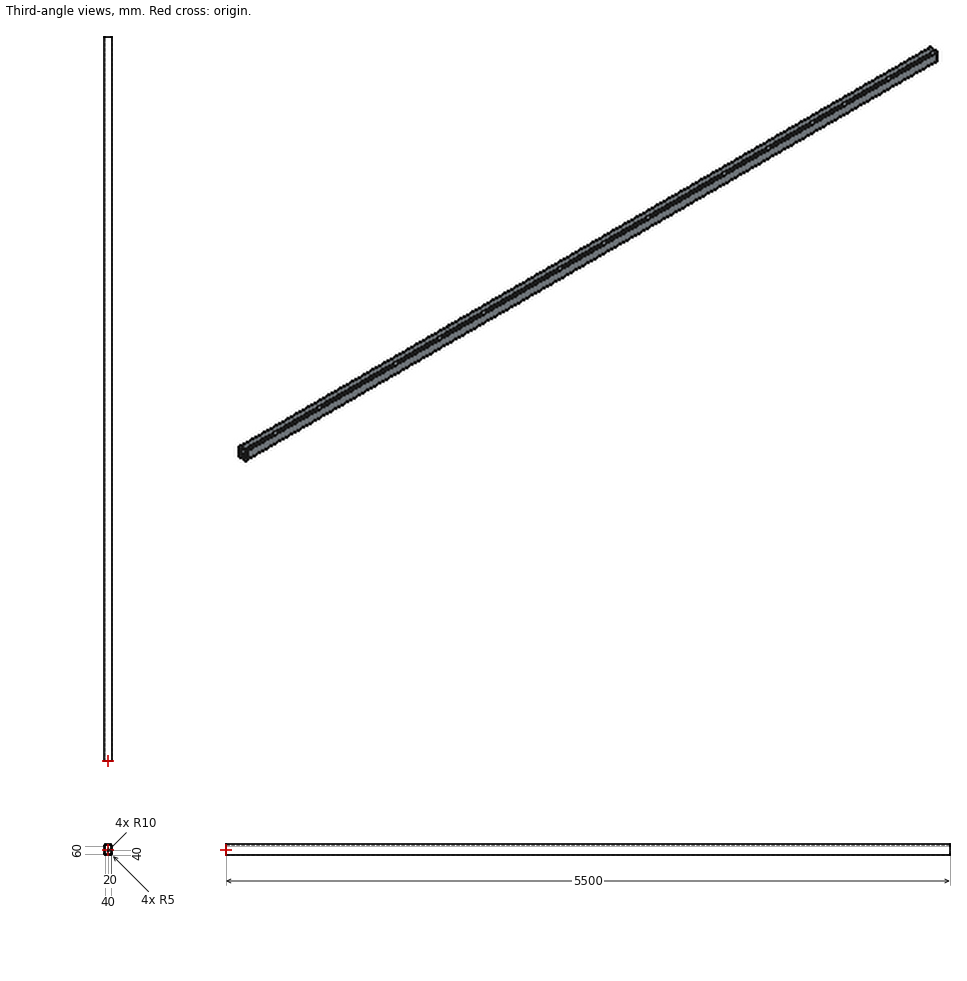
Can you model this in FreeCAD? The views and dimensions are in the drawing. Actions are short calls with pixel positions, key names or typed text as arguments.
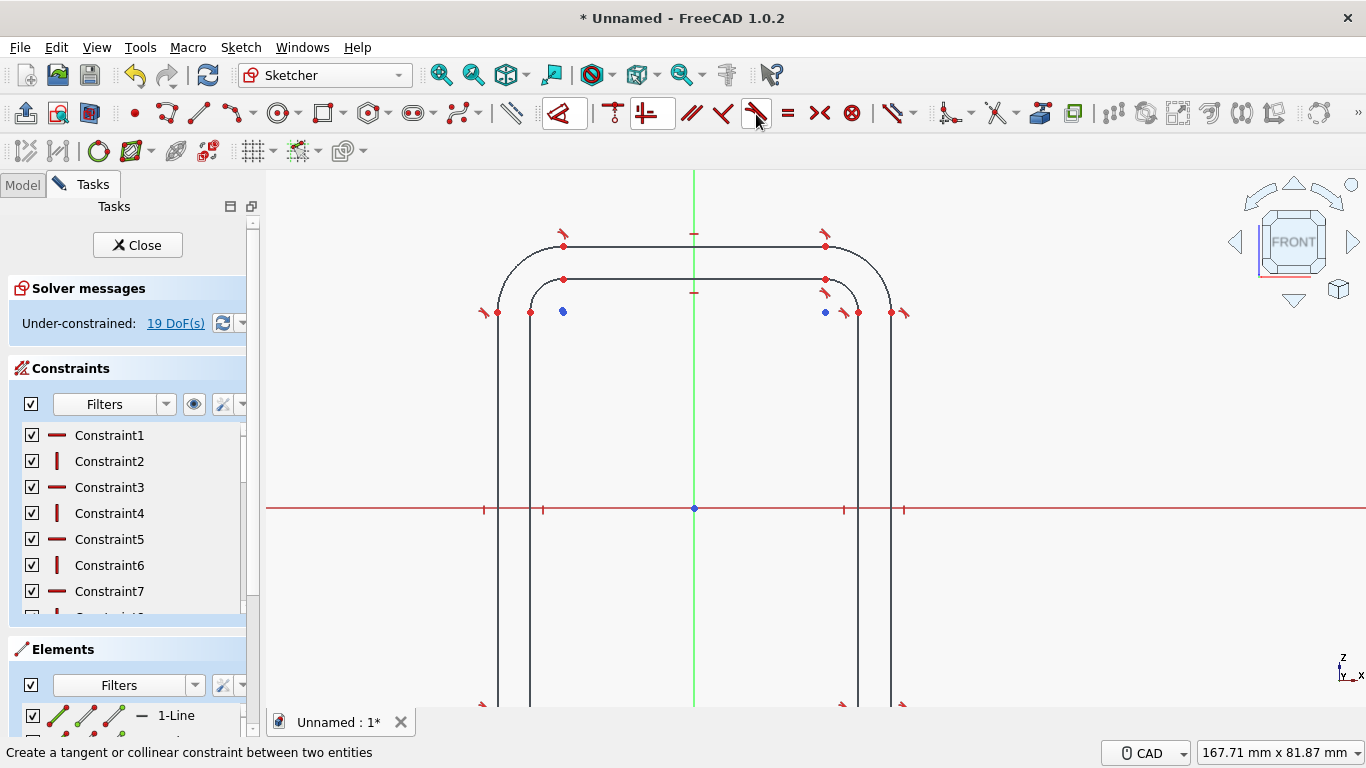
click(747, 279)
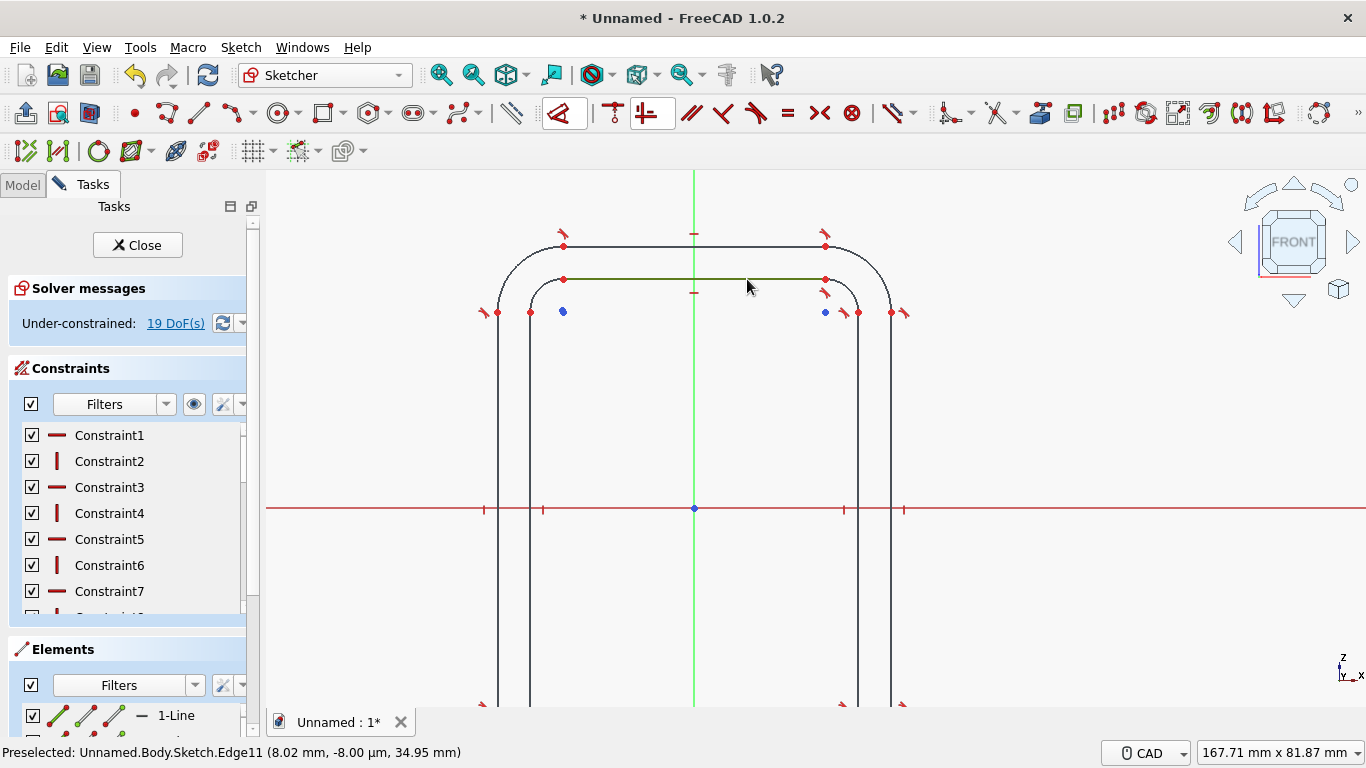
click(548, 282)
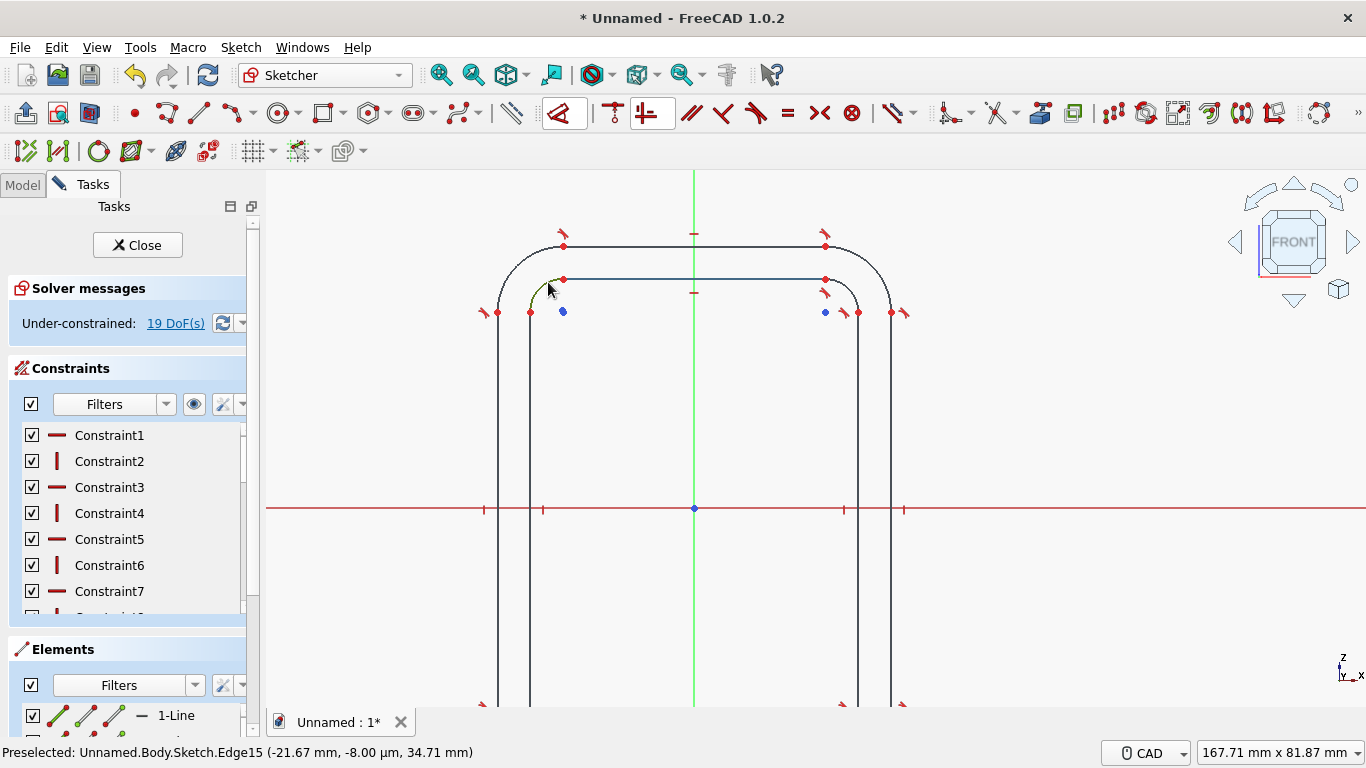
click(756, 114)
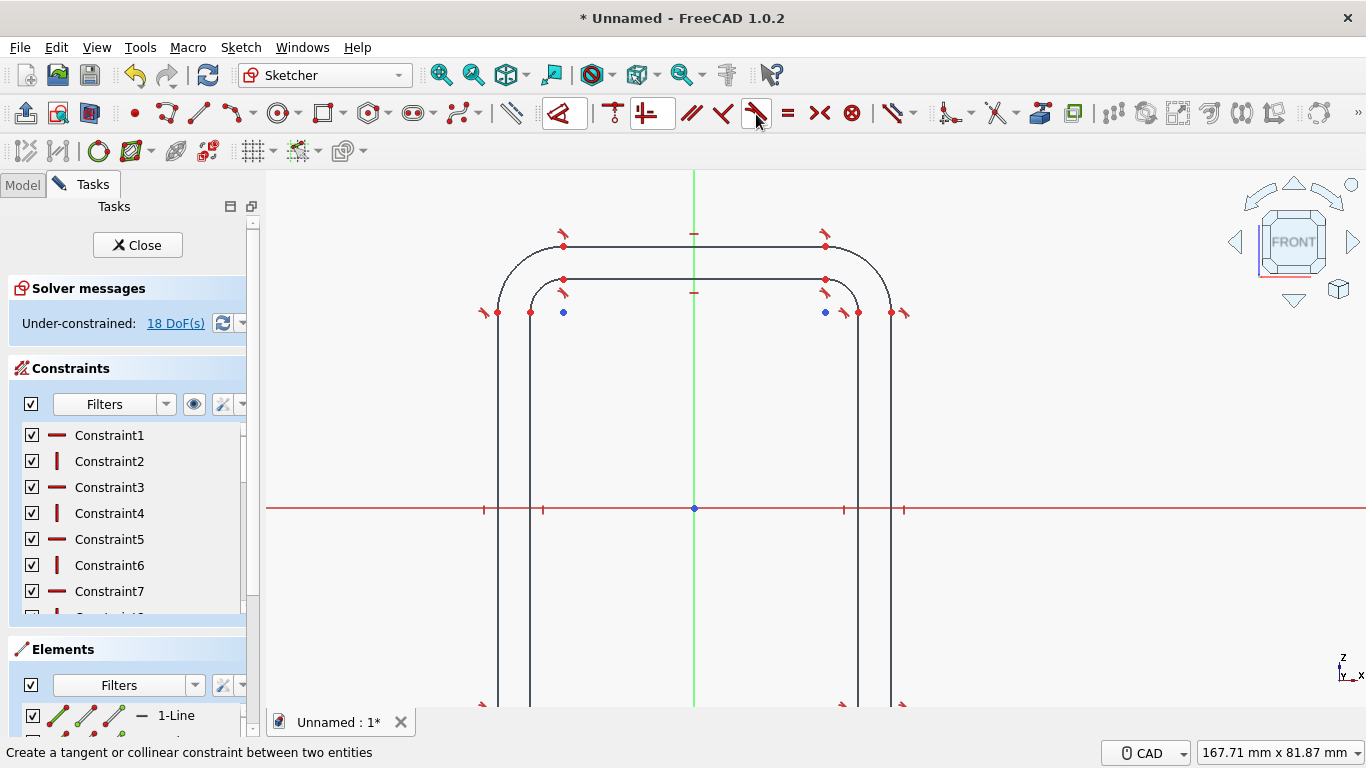
click(530, 431)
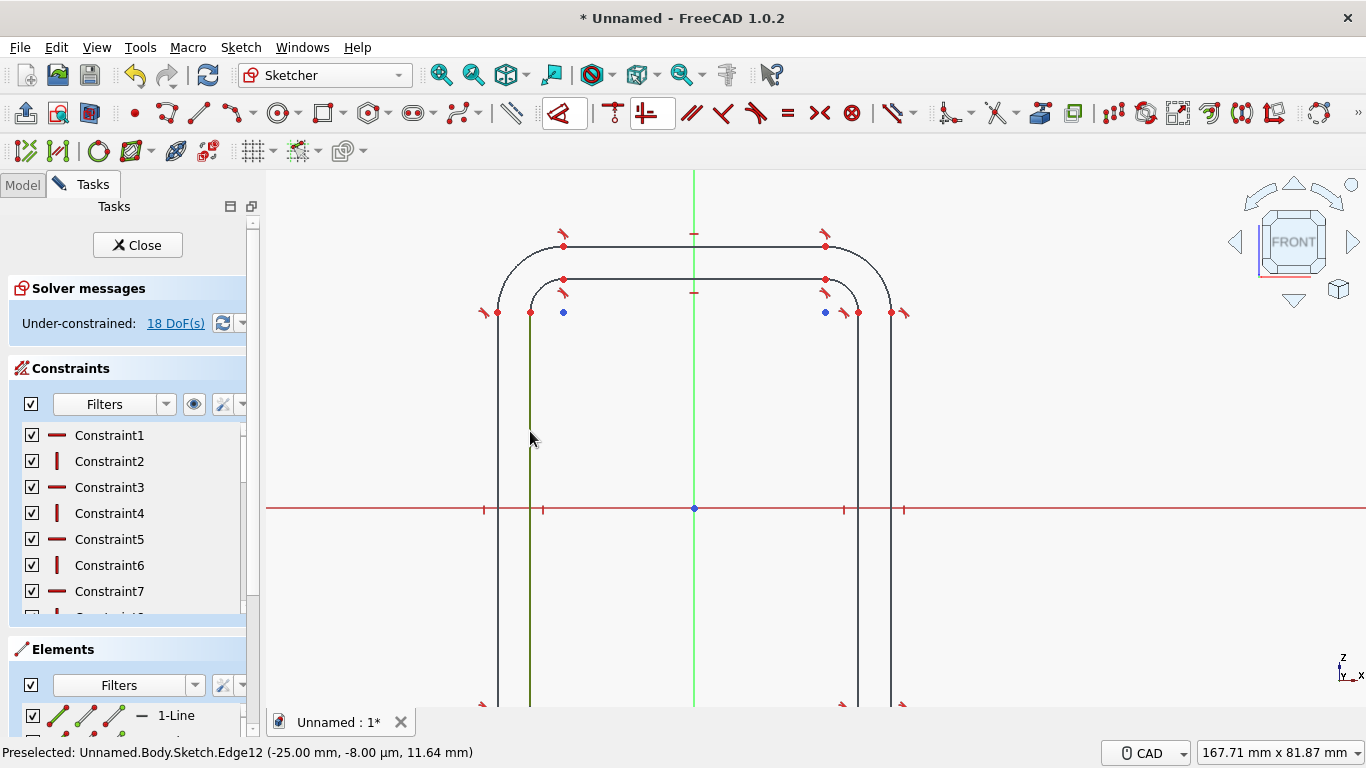
click(549, 283)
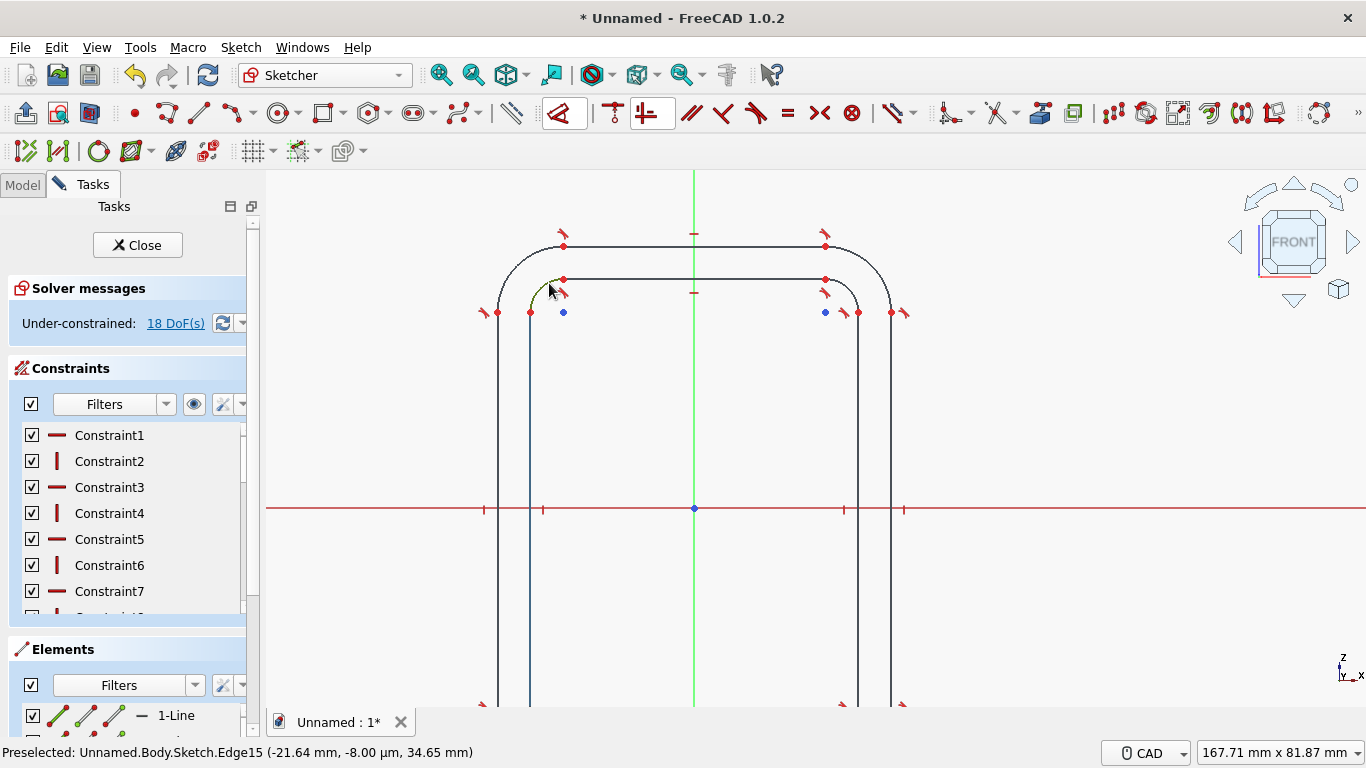
click(756, 114)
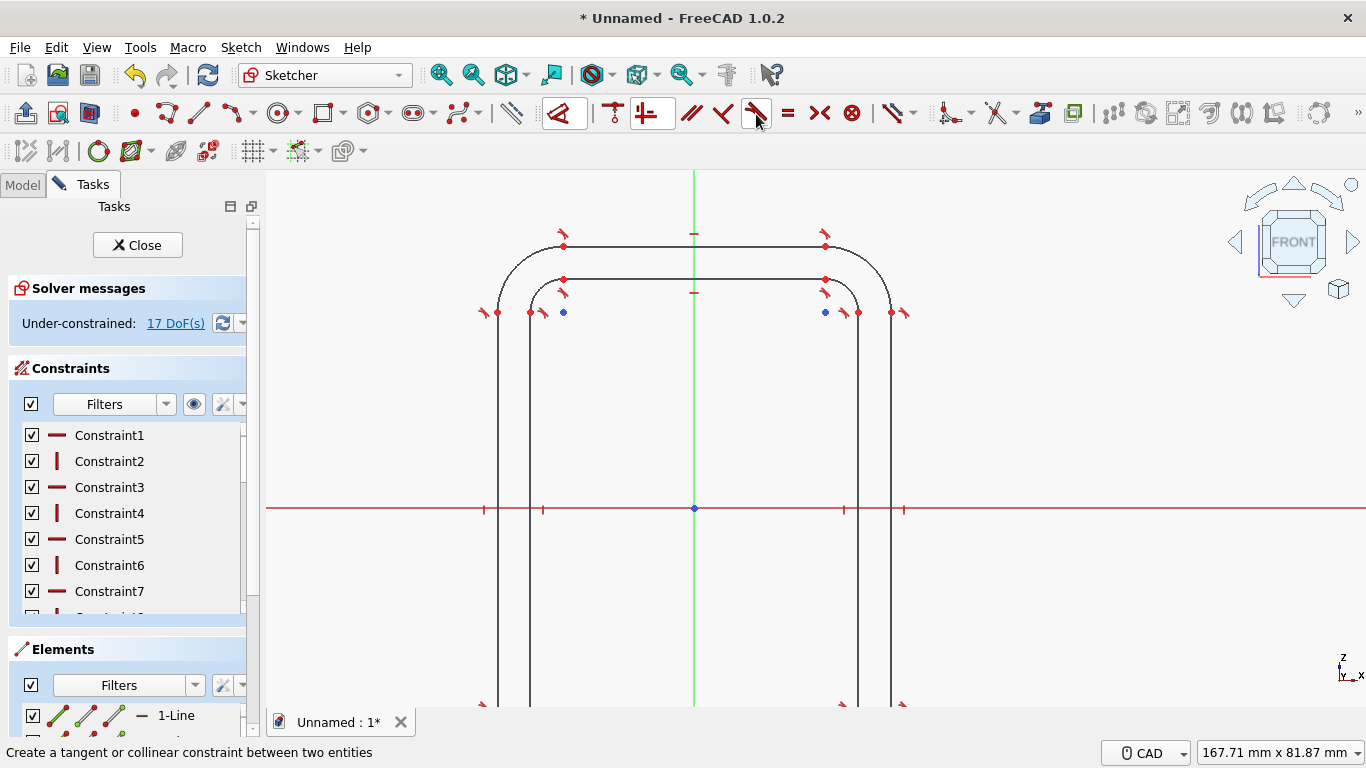
click(530, 431)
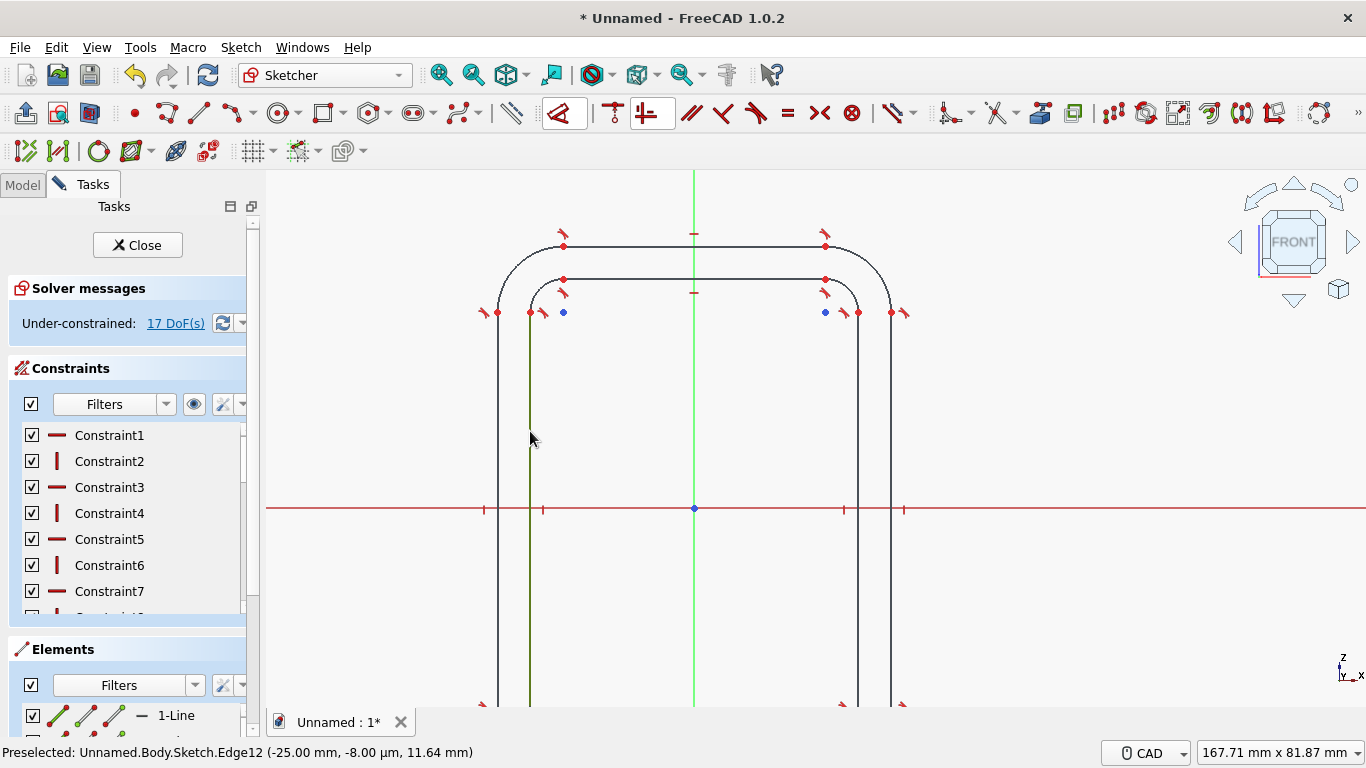
scroll(855, 297, down, 2)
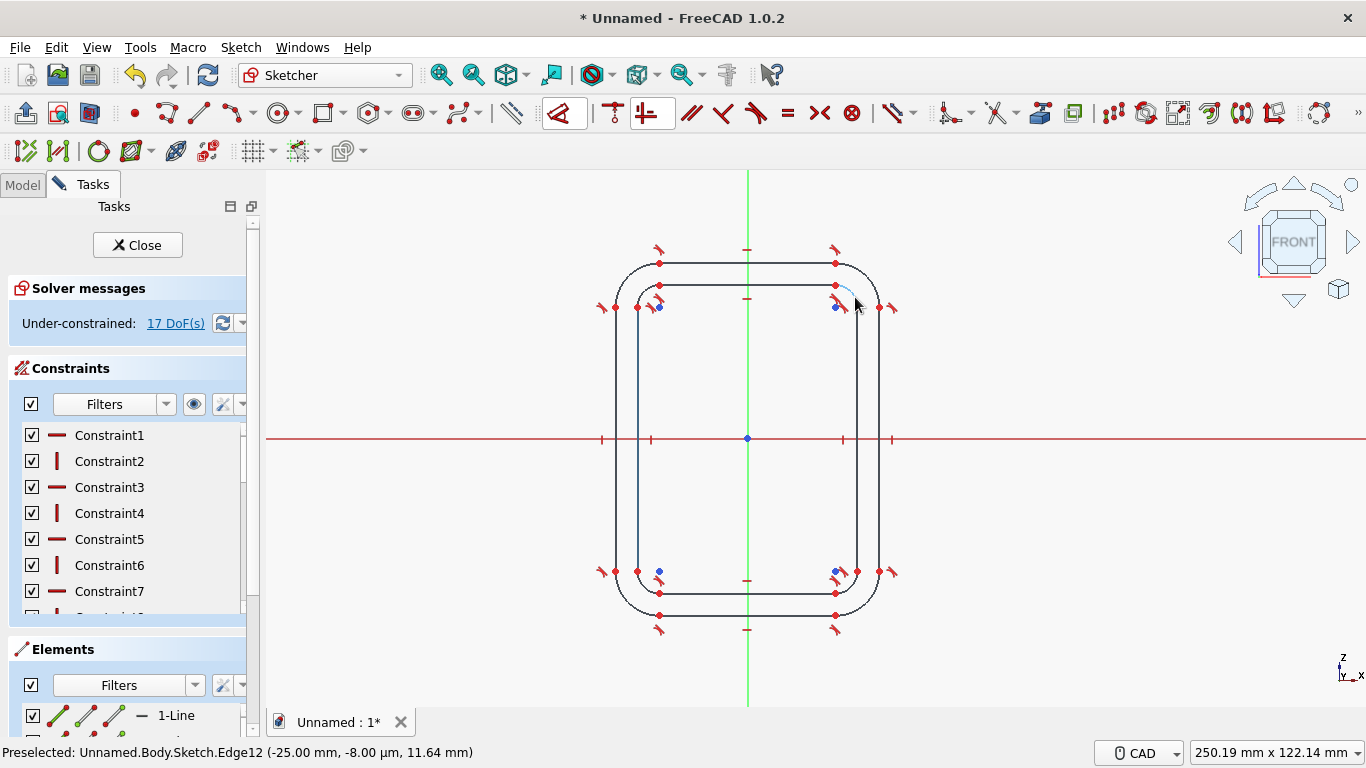
scroll(640, 582, up, 2)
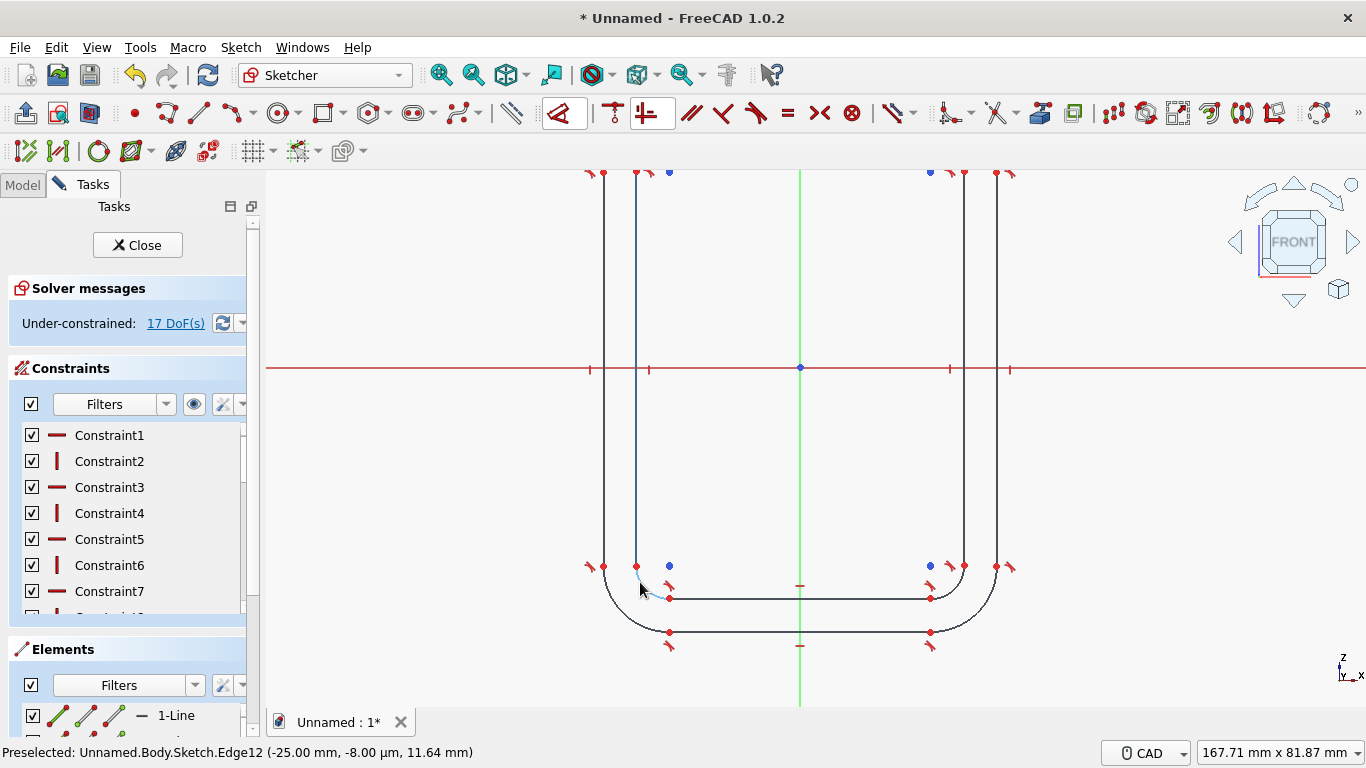
click(640, 581)